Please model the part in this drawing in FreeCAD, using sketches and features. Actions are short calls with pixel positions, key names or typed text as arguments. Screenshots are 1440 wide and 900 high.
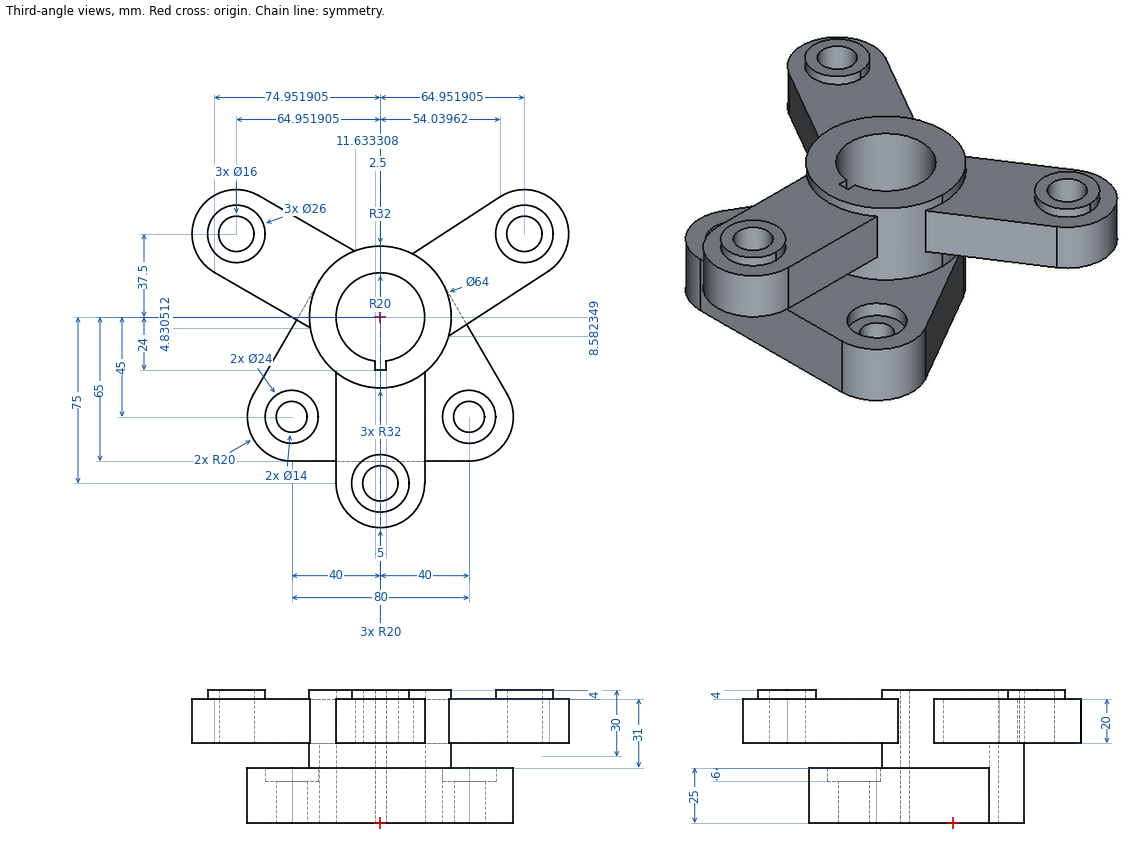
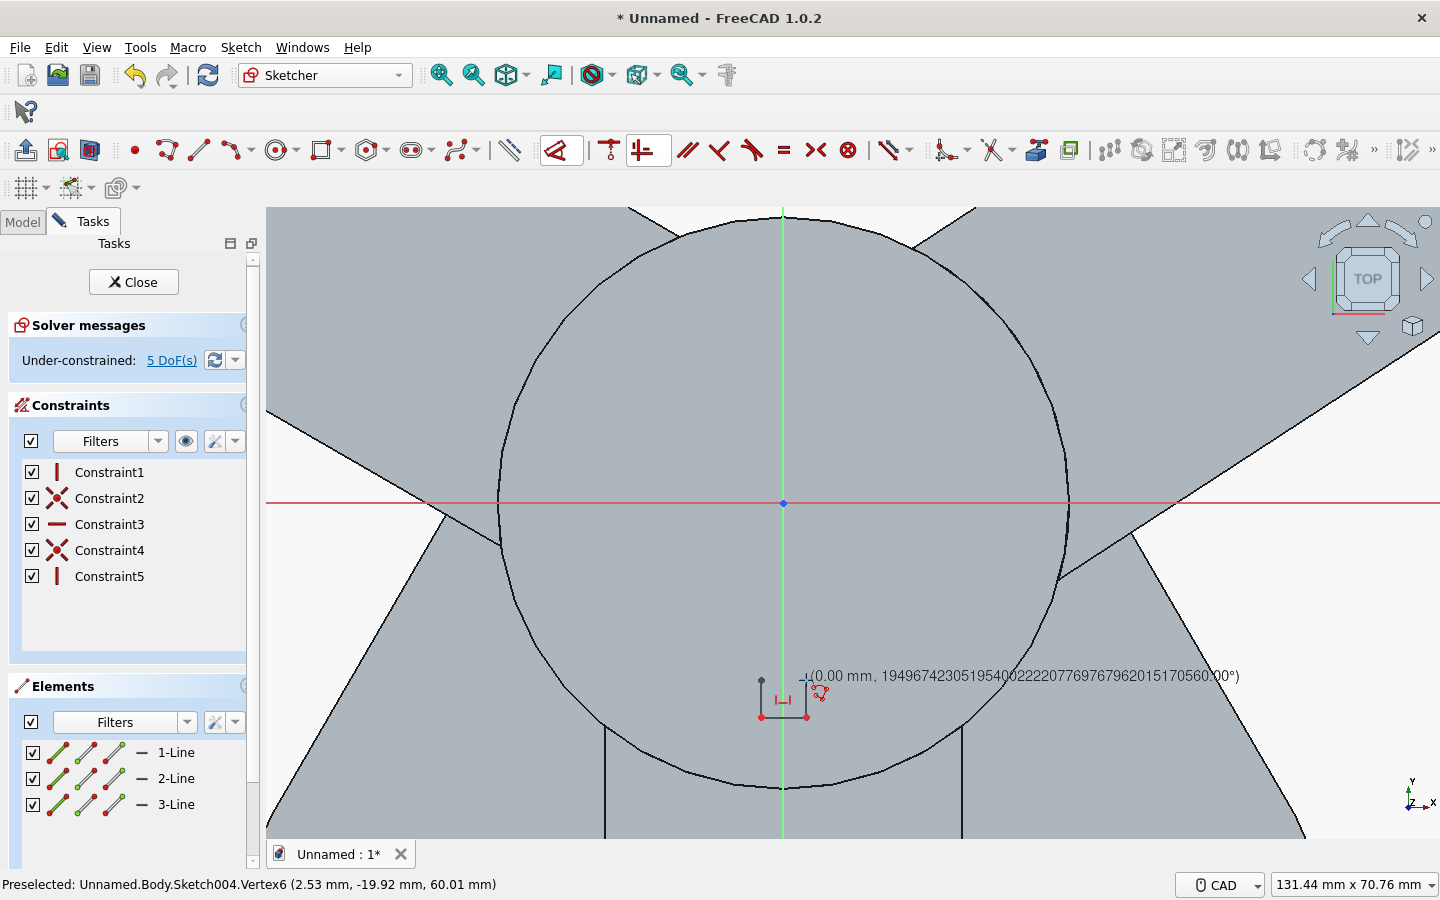
click(232, 150)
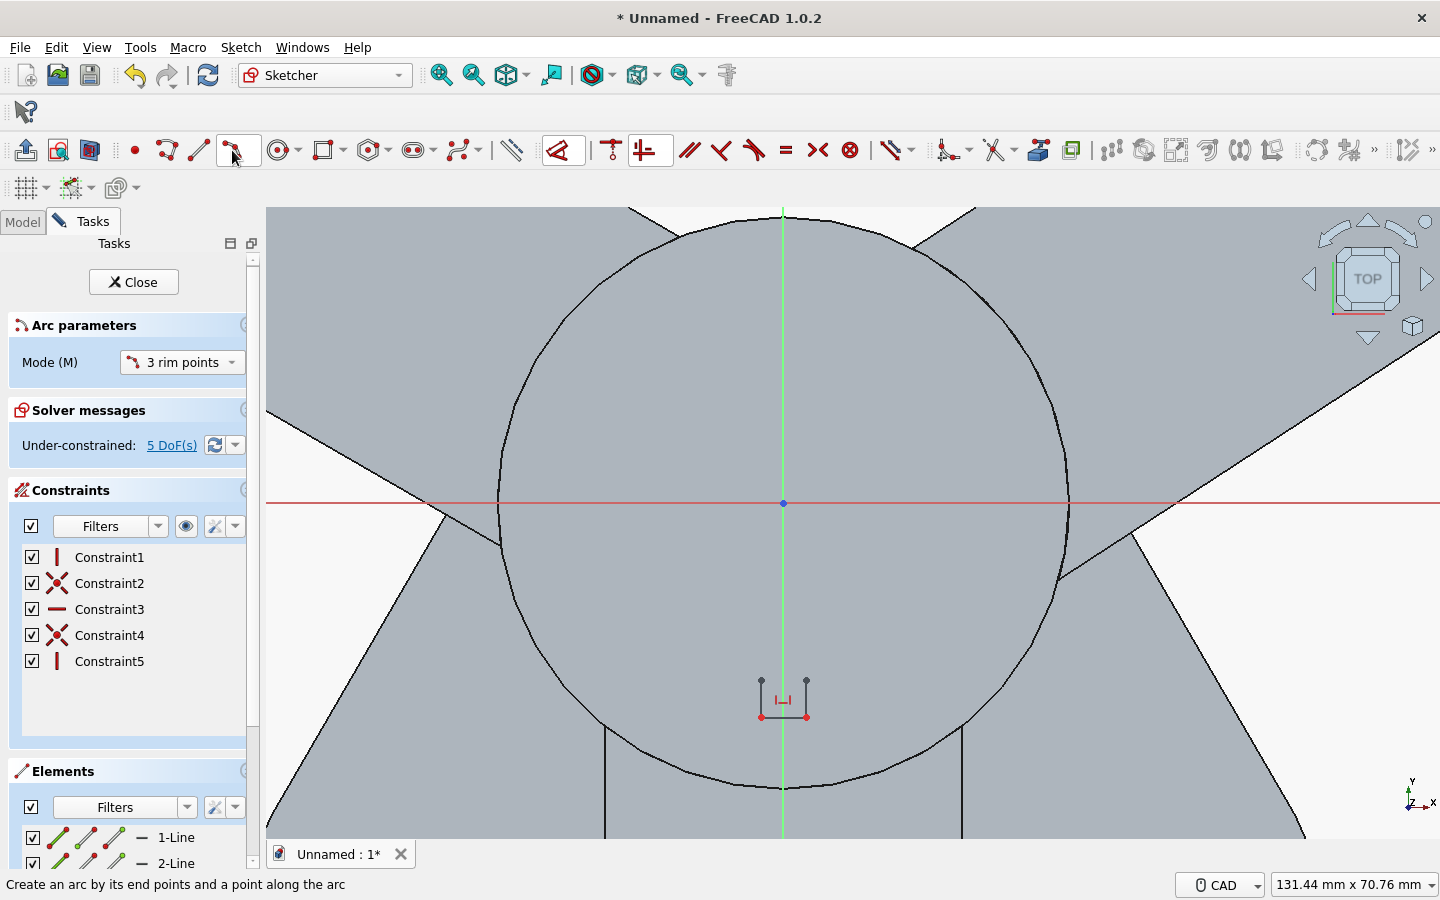
click(806, 681)
click(761, 681)
click(885, 356)
key(Escape)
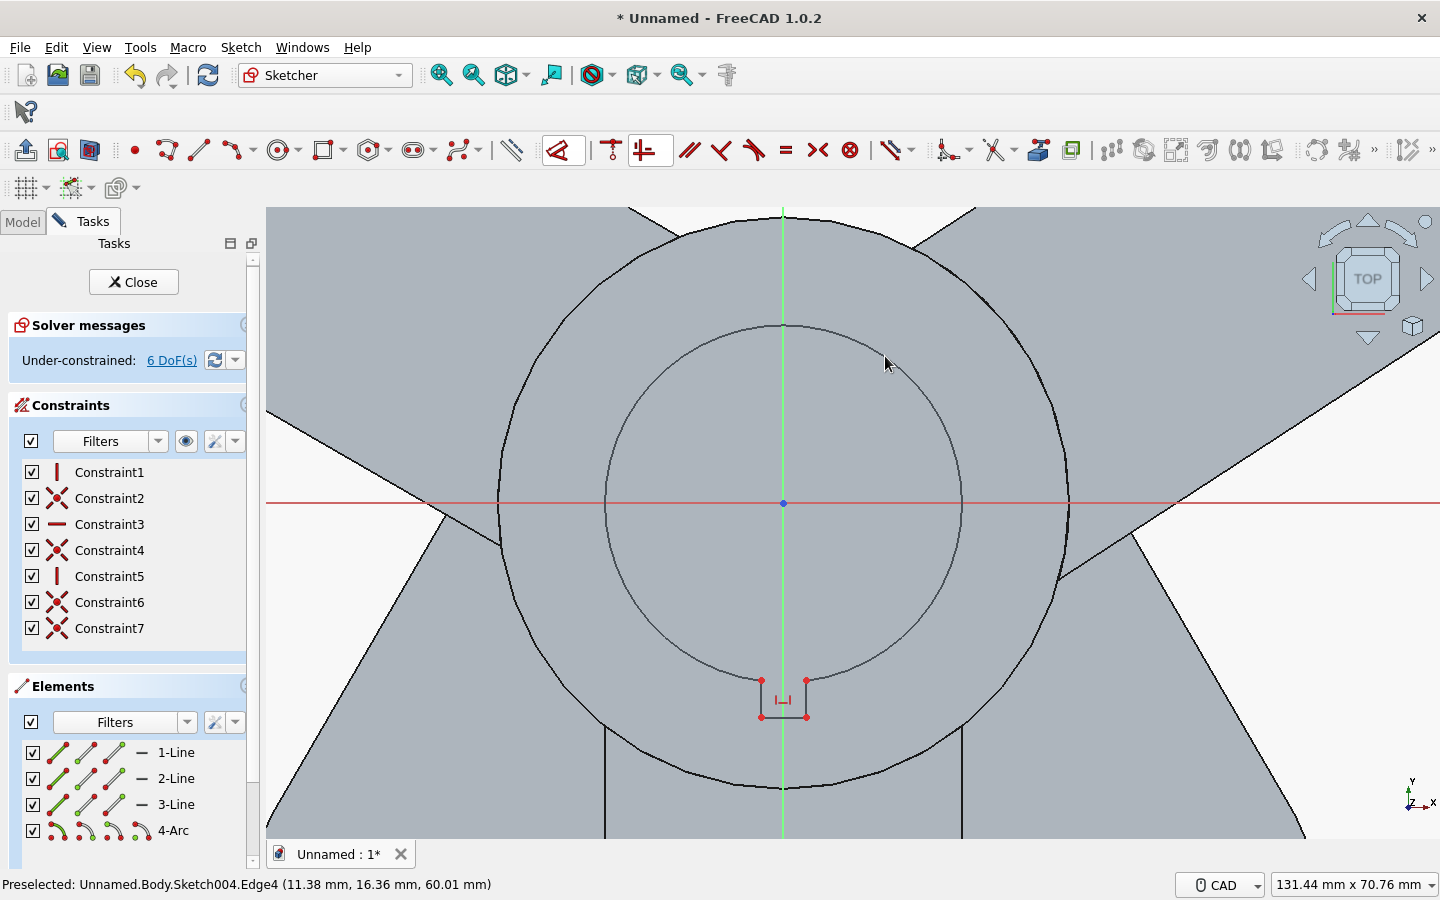
drag(773, 493, 794, 514)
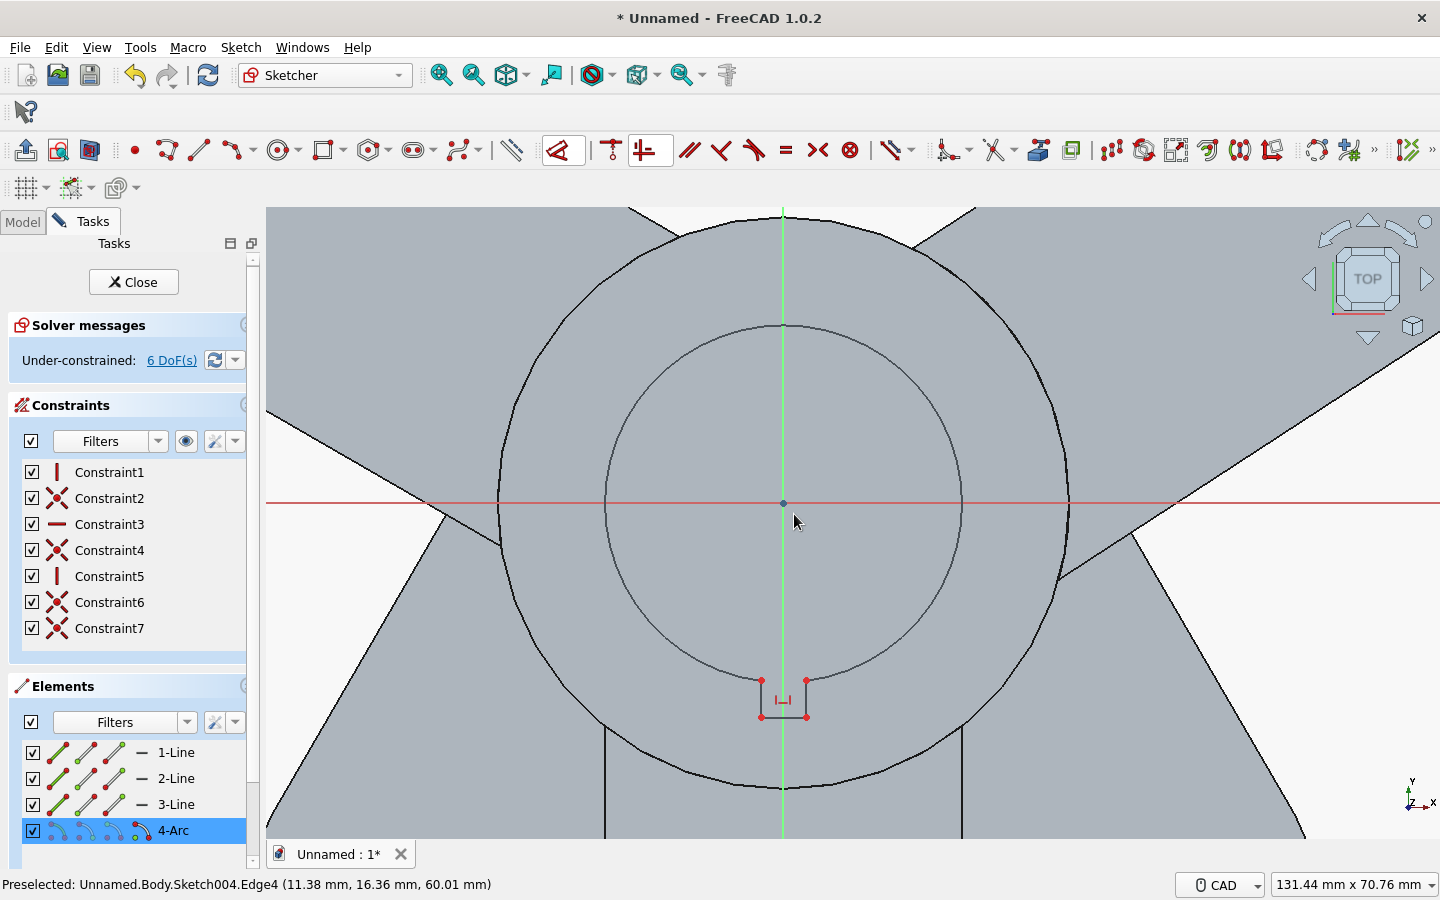
click(612, 150)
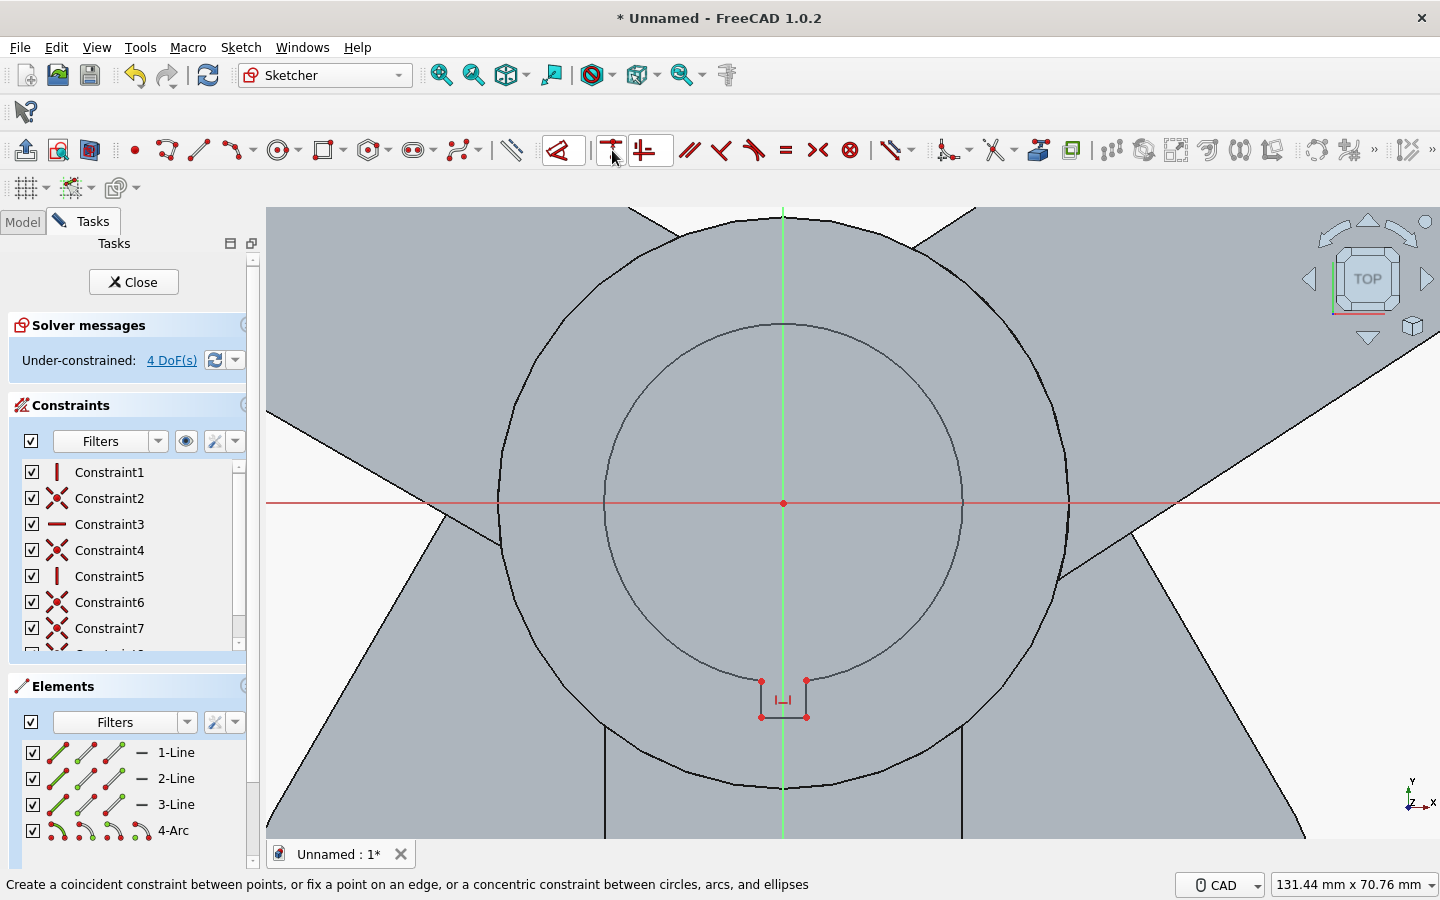
click(558, 150)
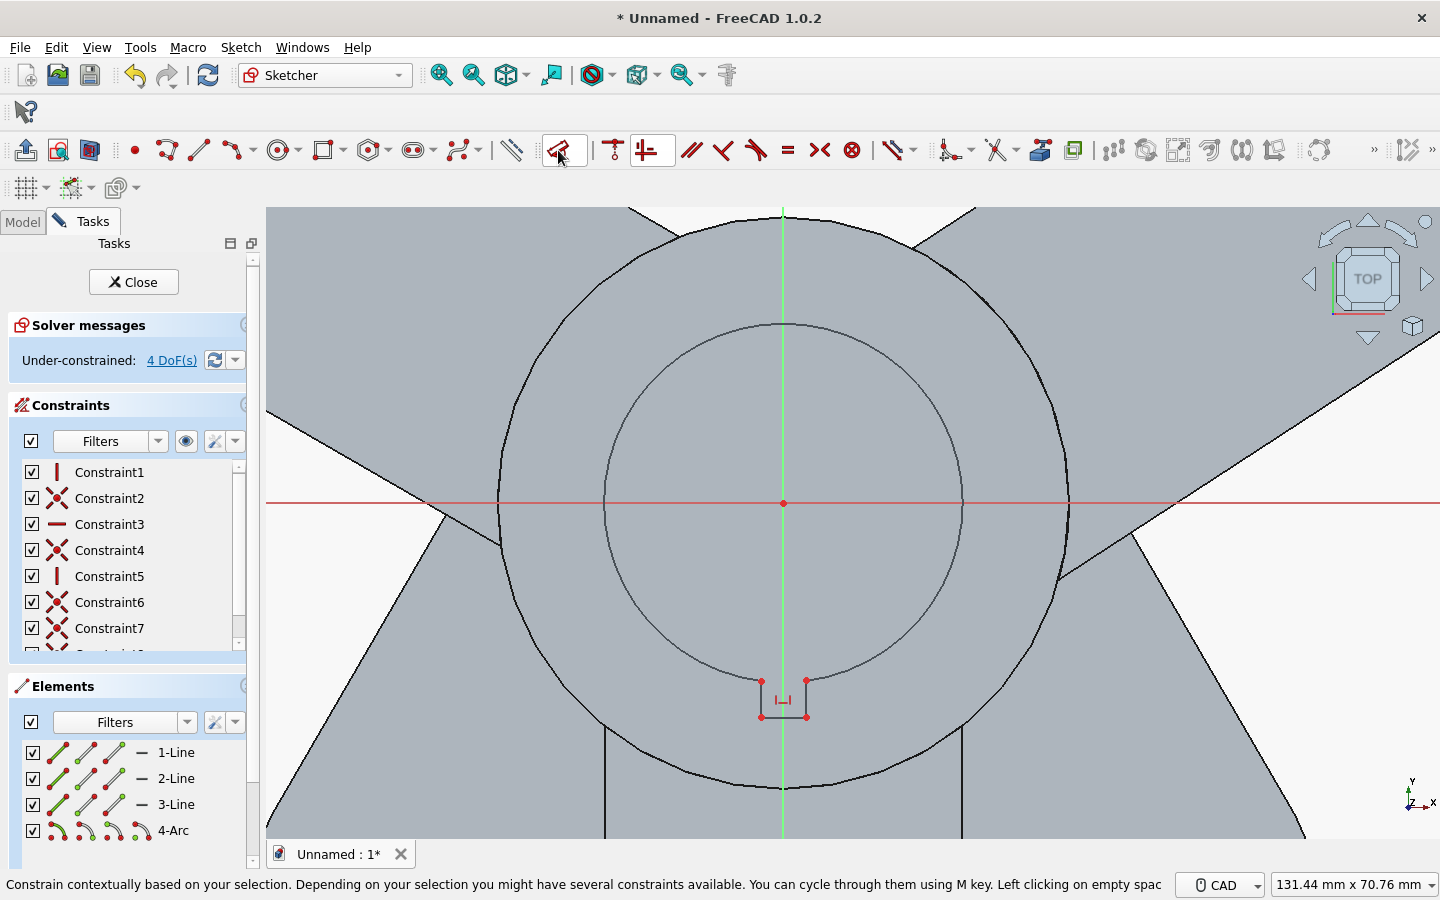
click(951, 439)
click(981, 428)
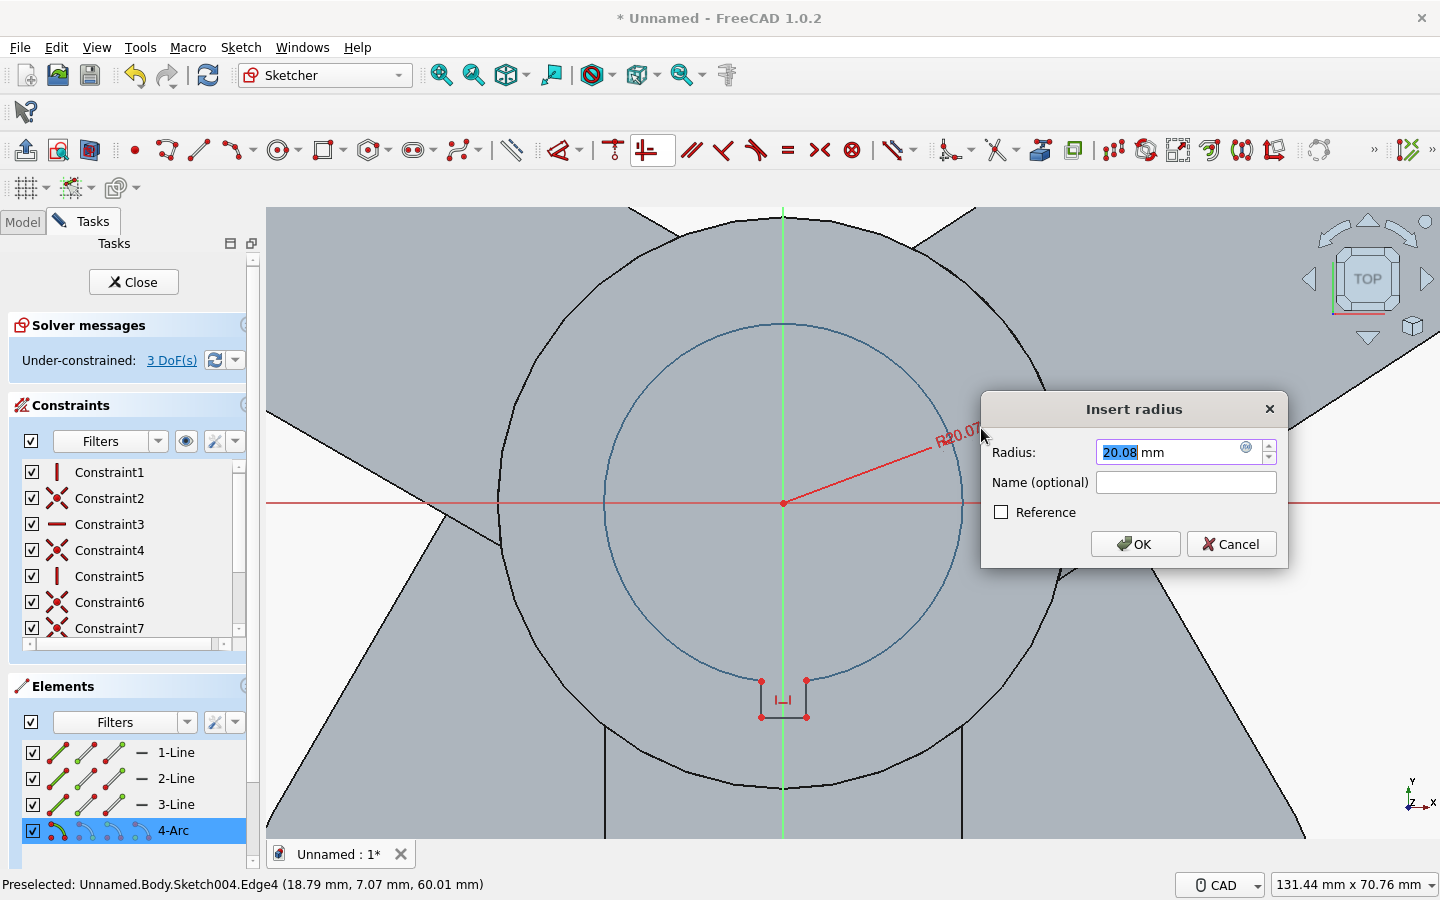
text(20)
key(Return)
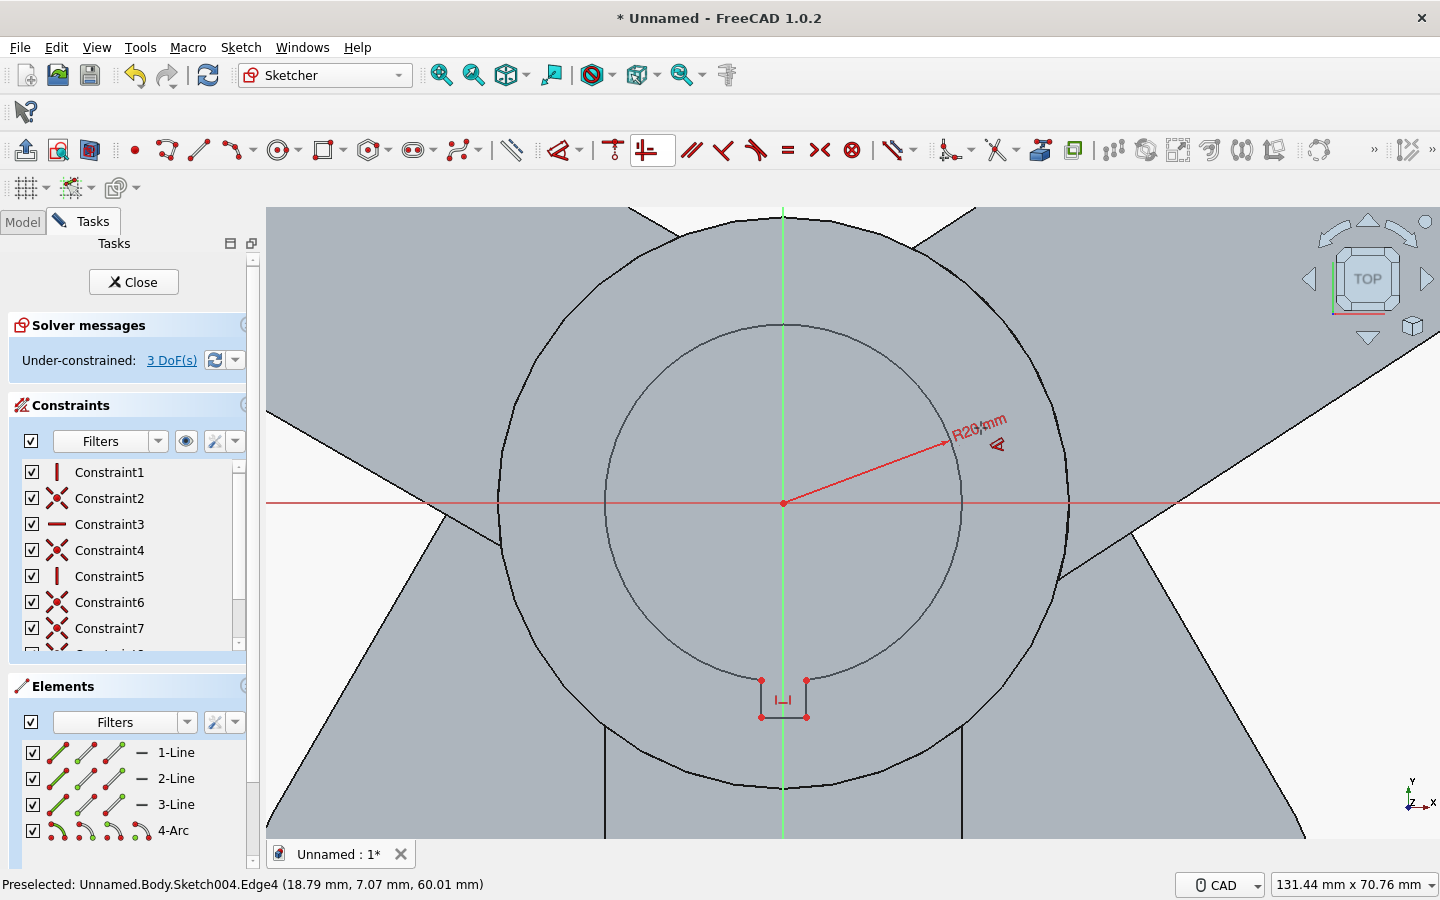
scroll(793, 718, up, 3)